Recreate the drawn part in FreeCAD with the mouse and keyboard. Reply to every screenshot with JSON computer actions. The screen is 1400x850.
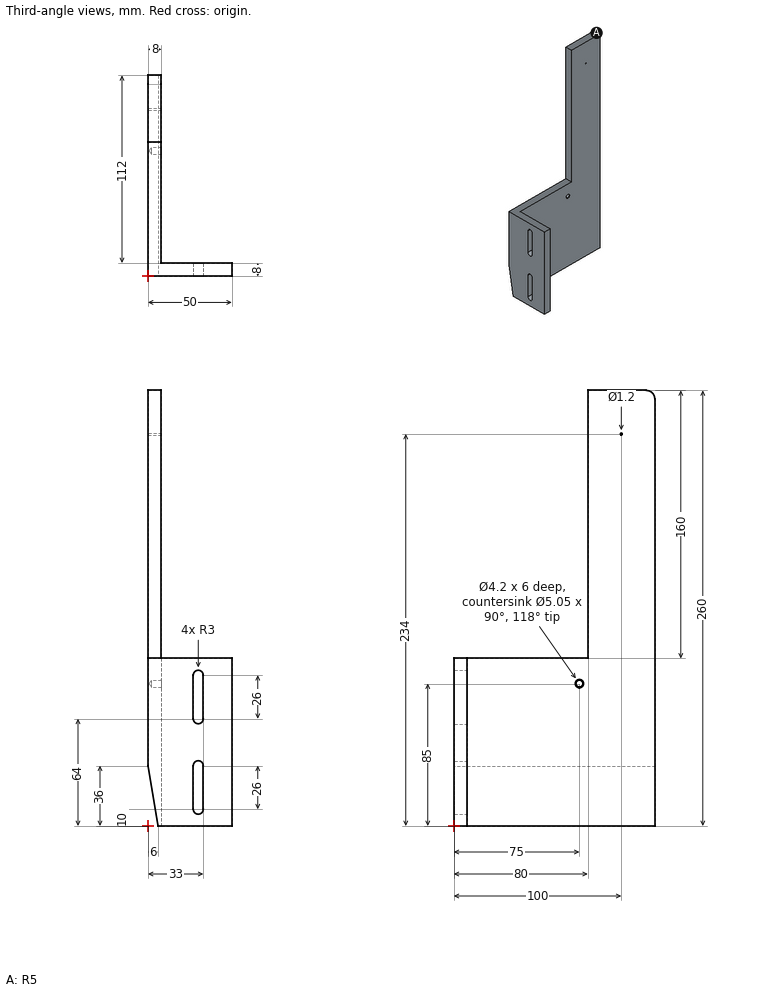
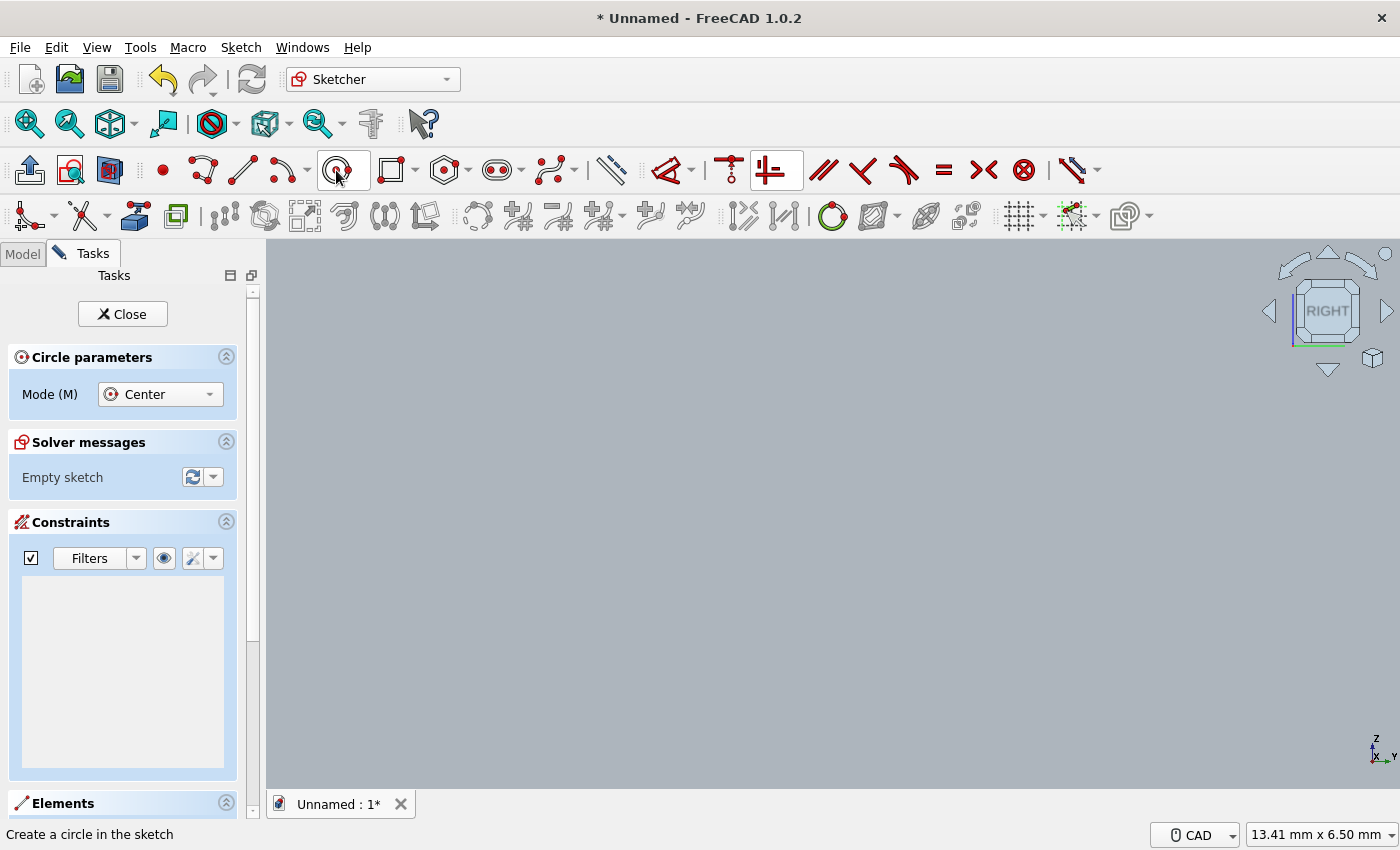
{"action": "left_click", "coordinate": [764, 514]}
{"action": "mouse_move", "coordinate": [890, 388]}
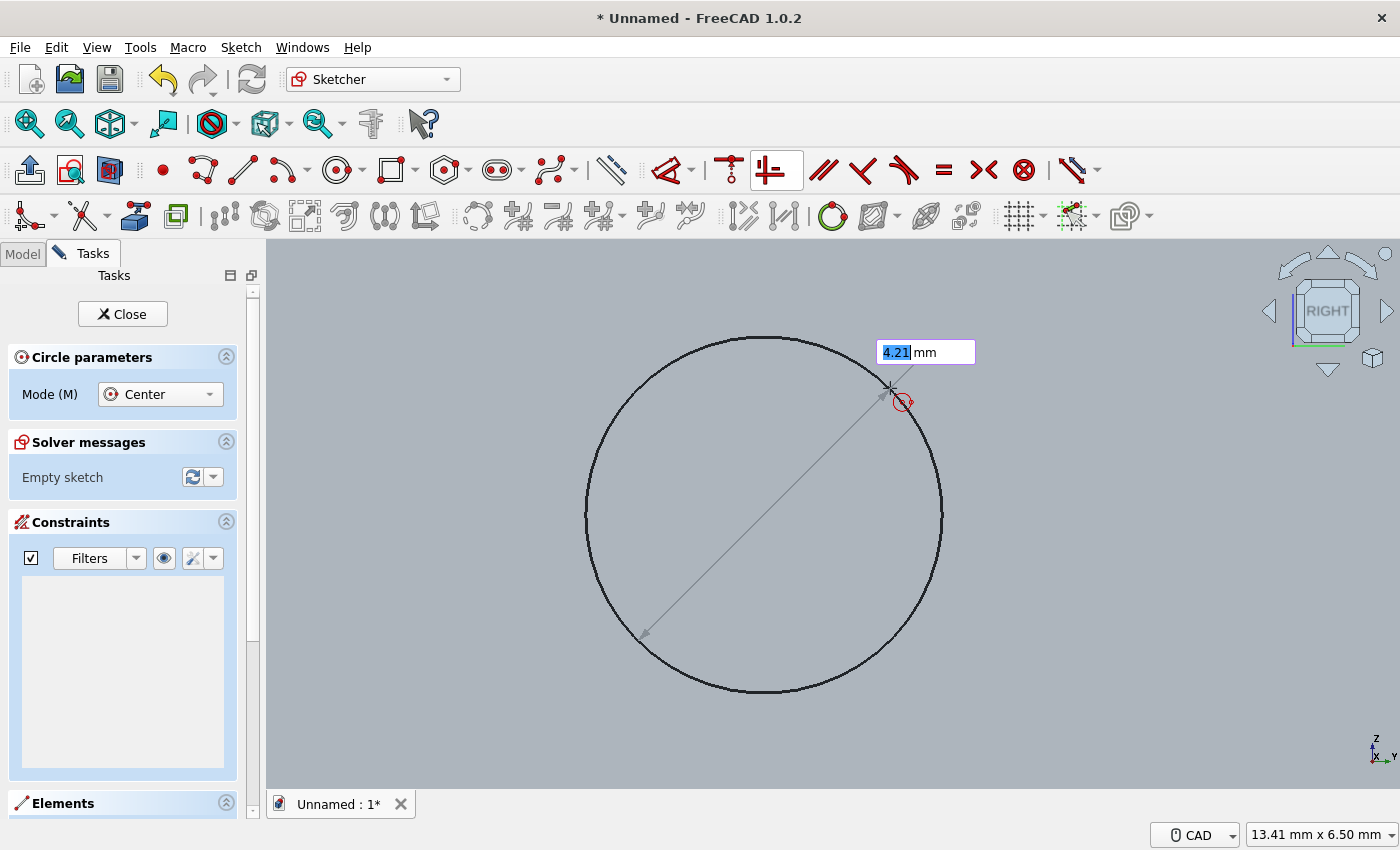
{"action": "type", "text": "4.2"}
{"action": "key", "text": "Return"}
{"action": "key", "text": "Escape"}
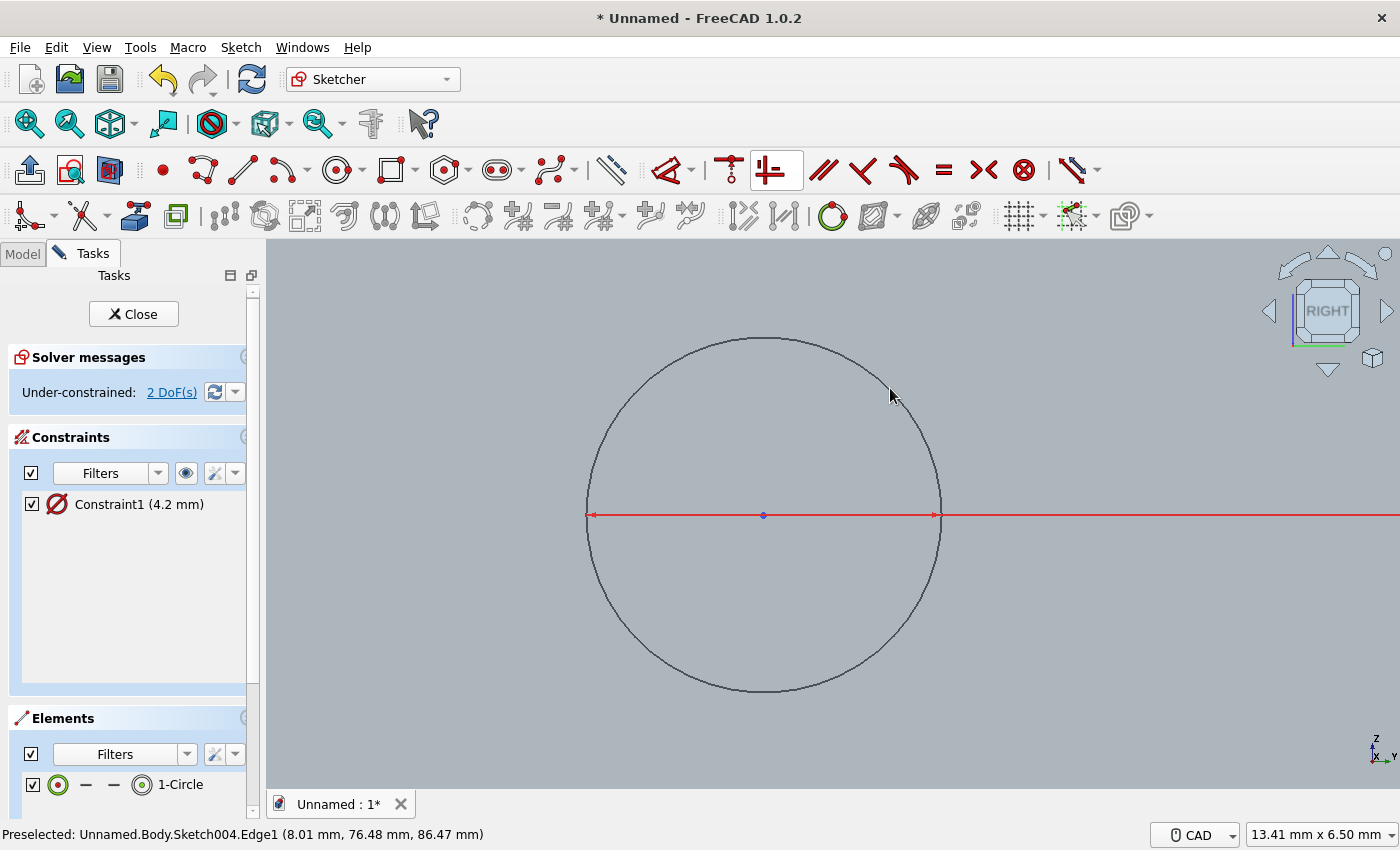
{"action": "left_click", "coordinate": [666, 170]}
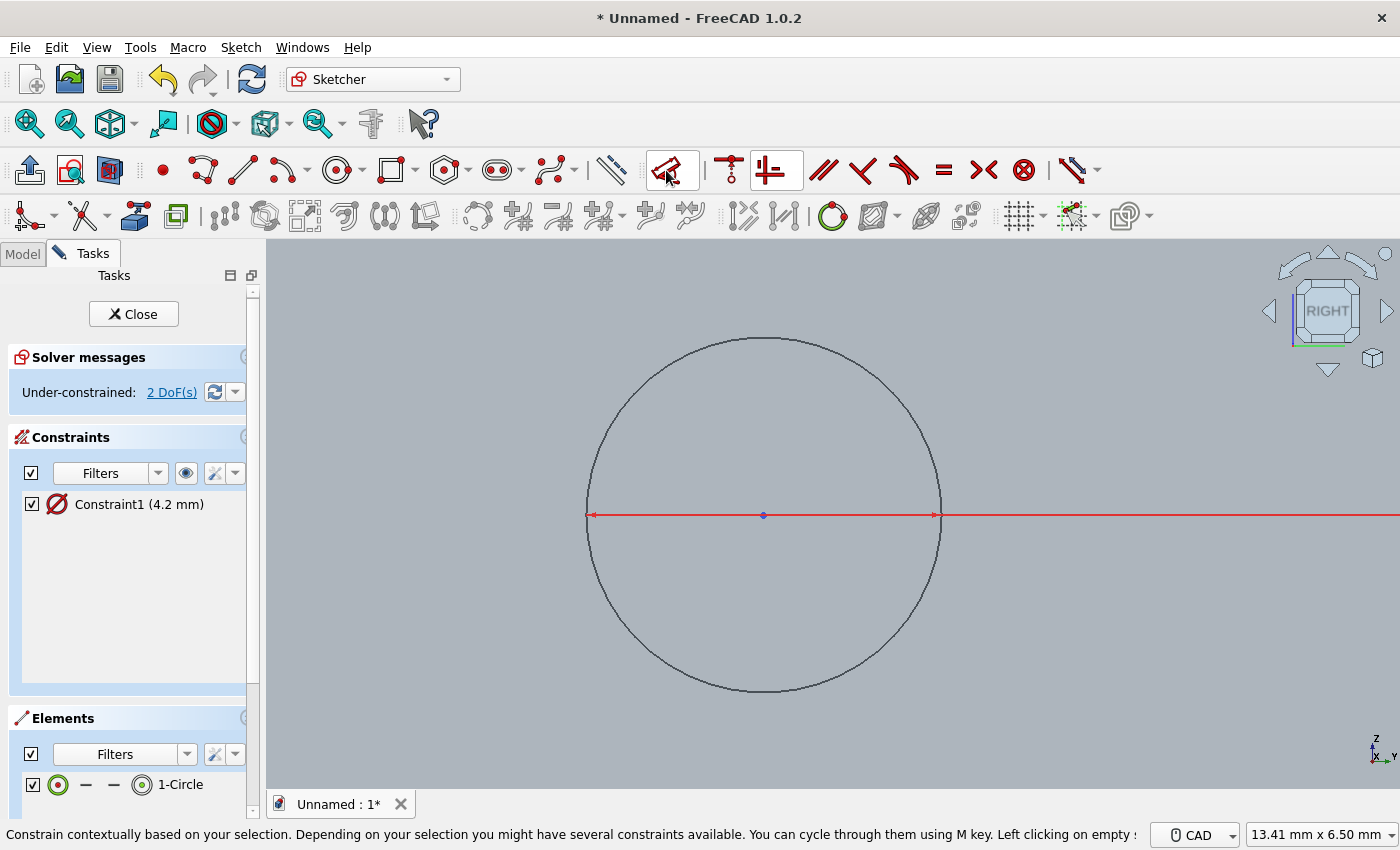
{"action": "left_click", "coordinate": [764, 515]}
{"action": "left_click", "coordinate": [529, 481]}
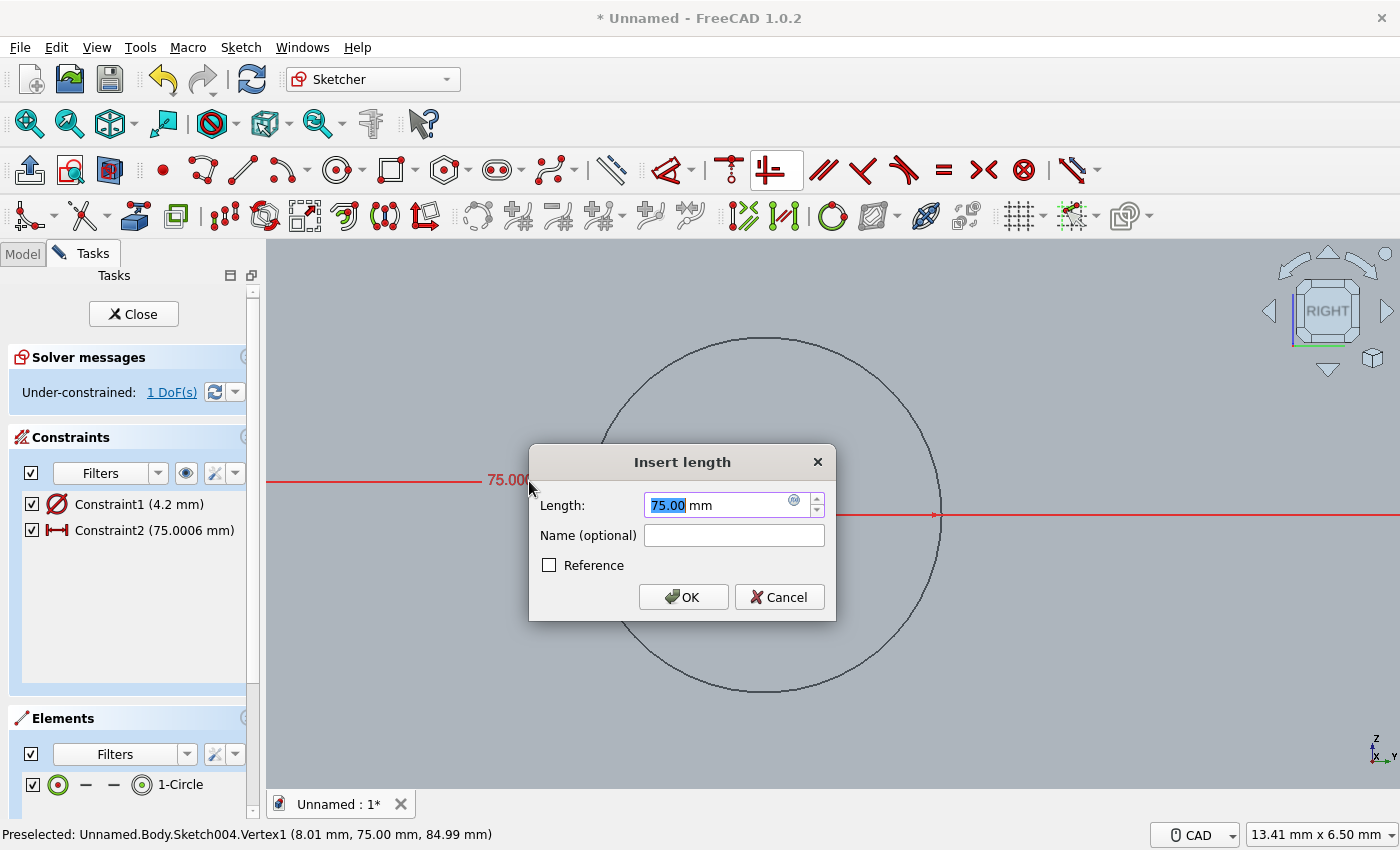
{"action": "type", "text": "75"}
{"action": "key", "text": "Return"}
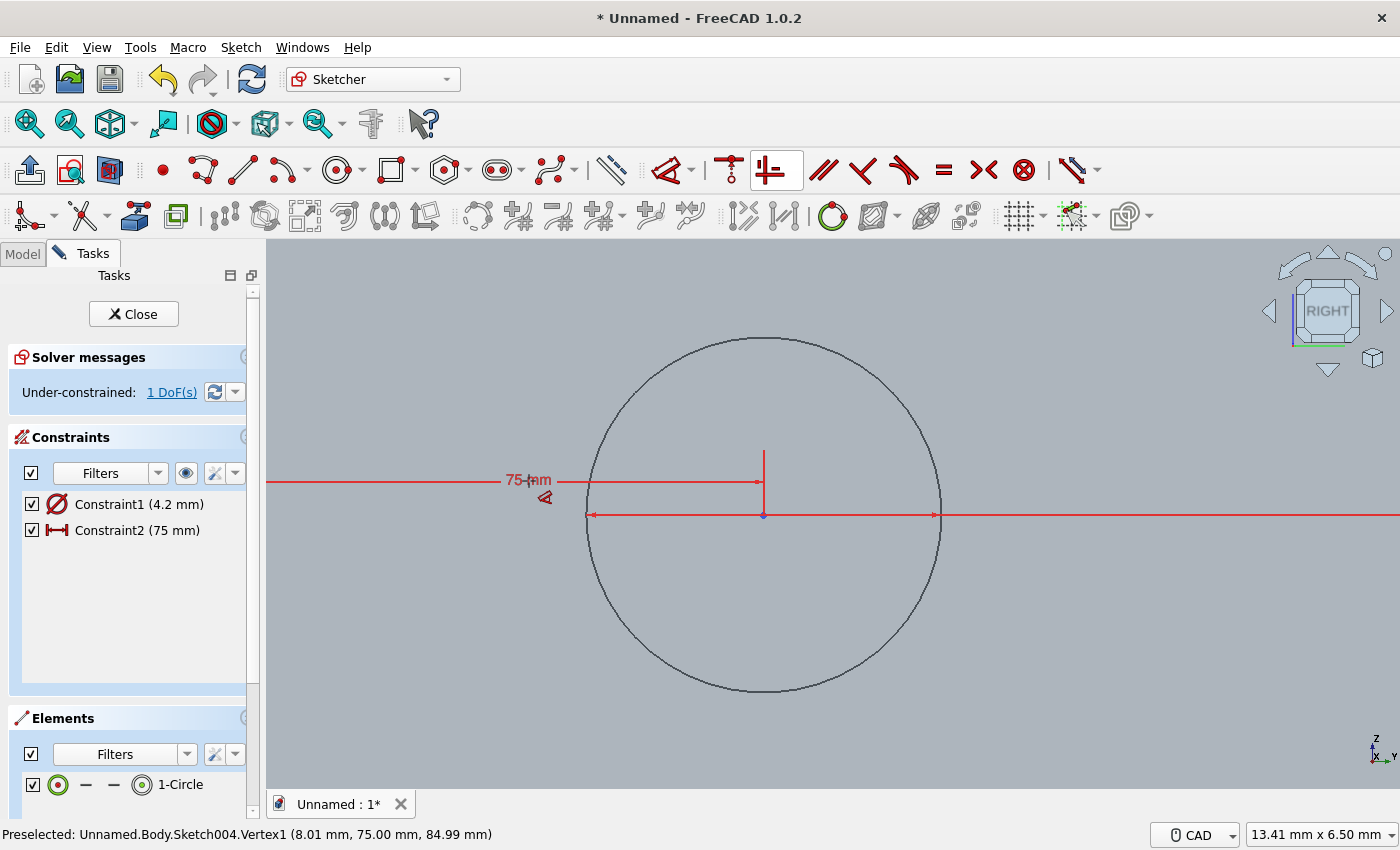
{"action": "left_click", "coordinate": [764, 515]}
{"action": "left_click", "coordinate": [798, 638]}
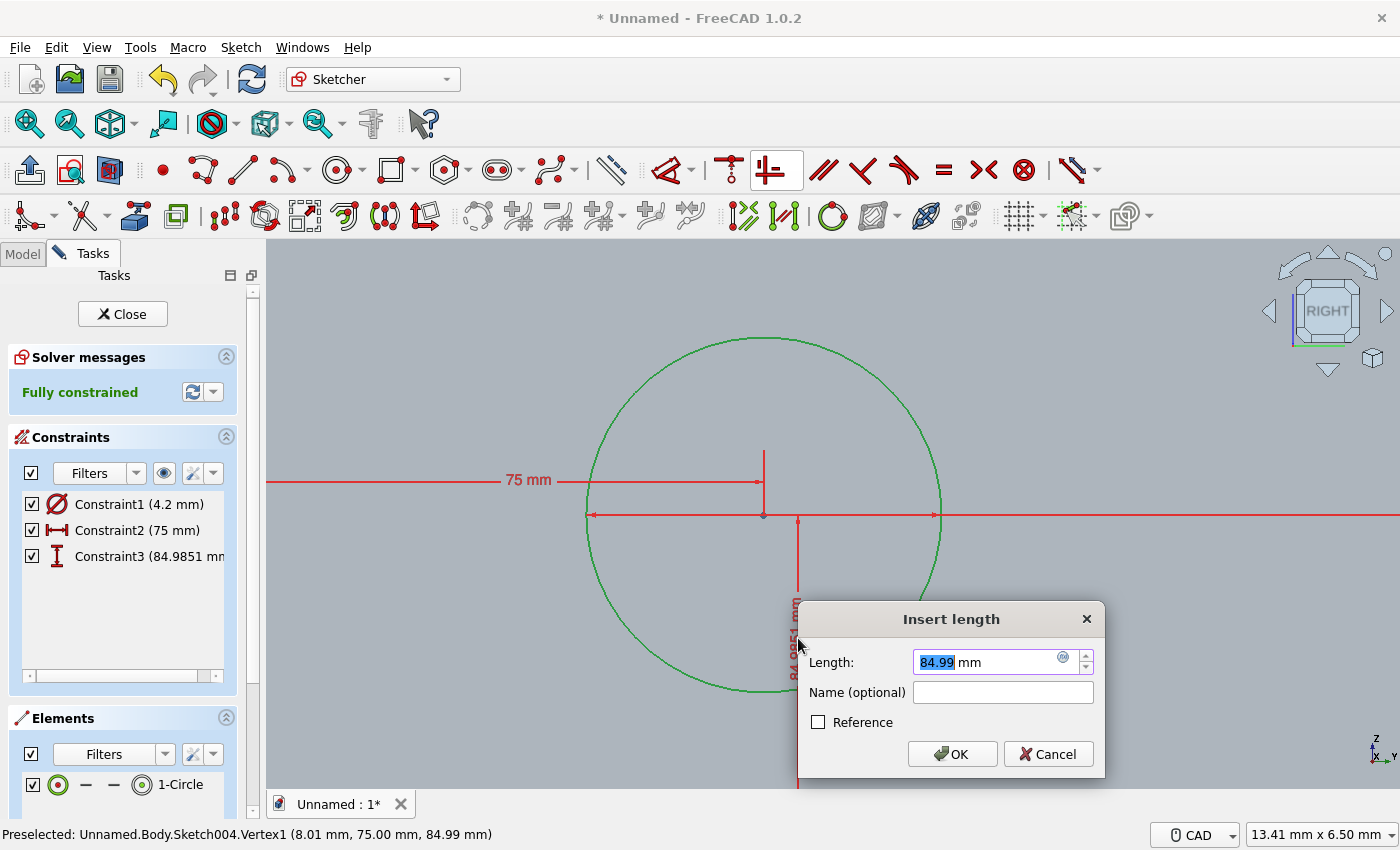
{"action": "type", "text": "85"}
{"action": "key", "text": "Return"}
{"action": "key", "text": "Escape"}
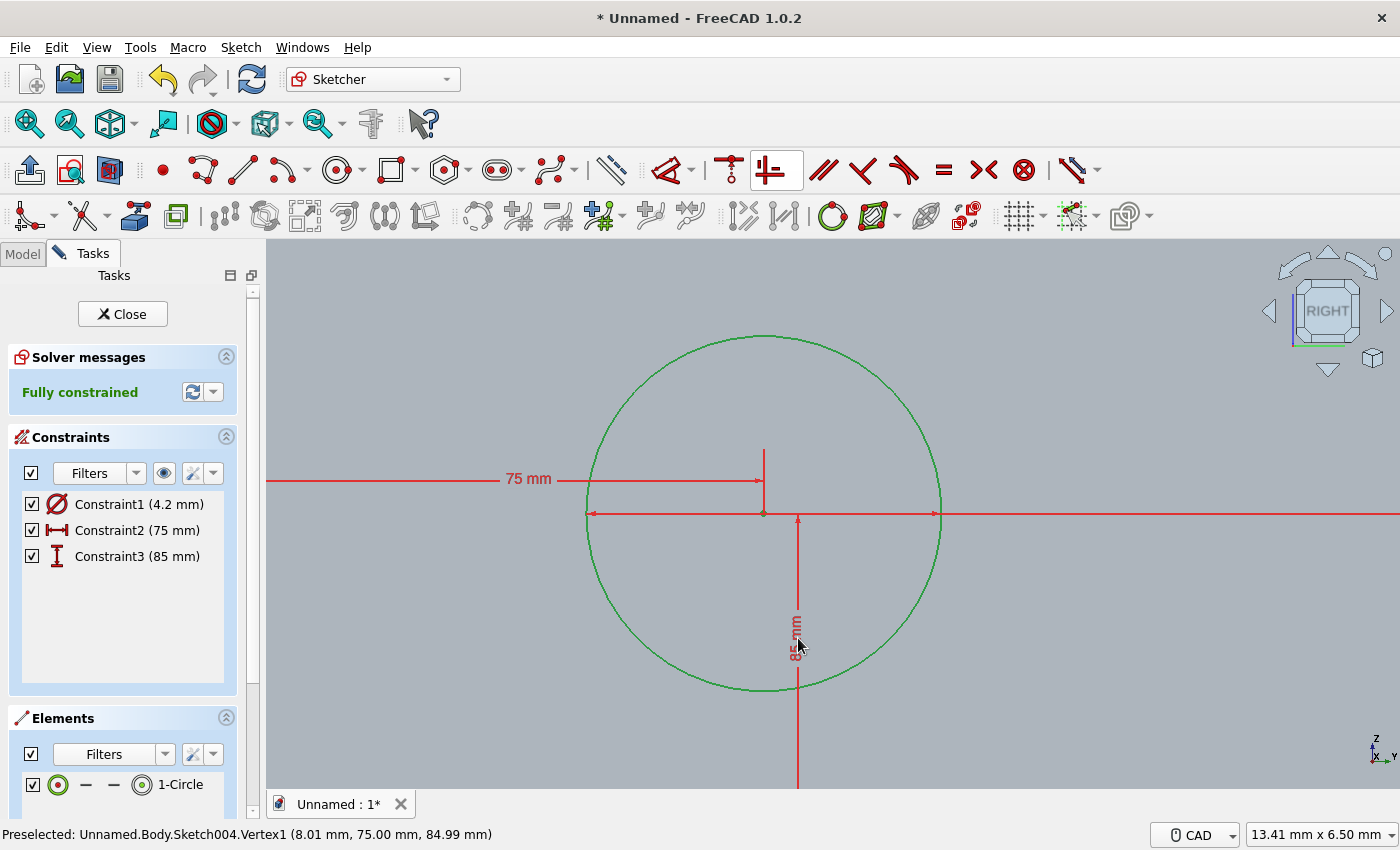
{"action": "left_click", "coordinate": [123, 314]}